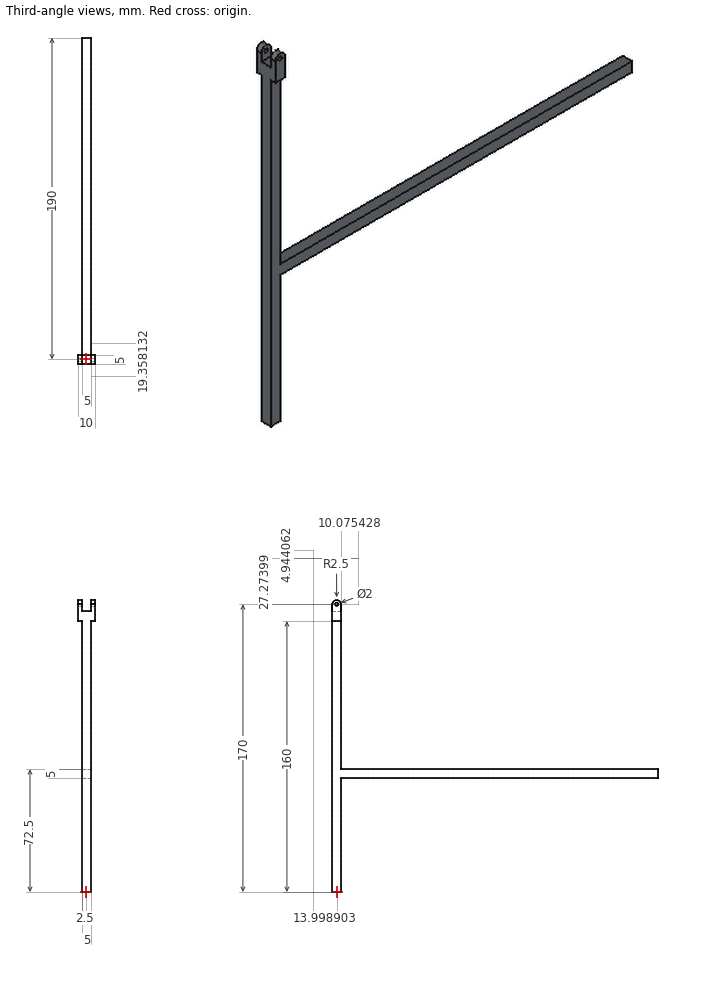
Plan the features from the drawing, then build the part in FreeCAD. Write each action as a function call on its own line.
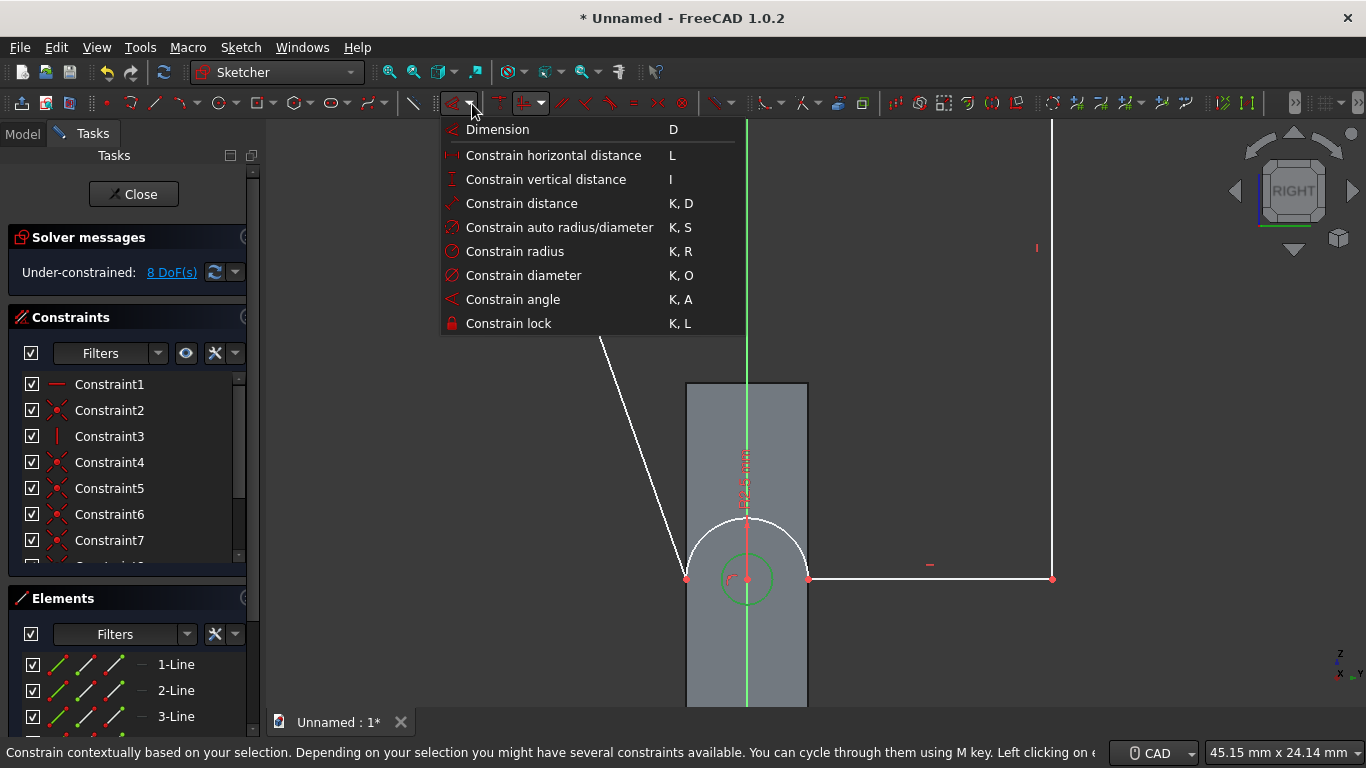
click(593, 275)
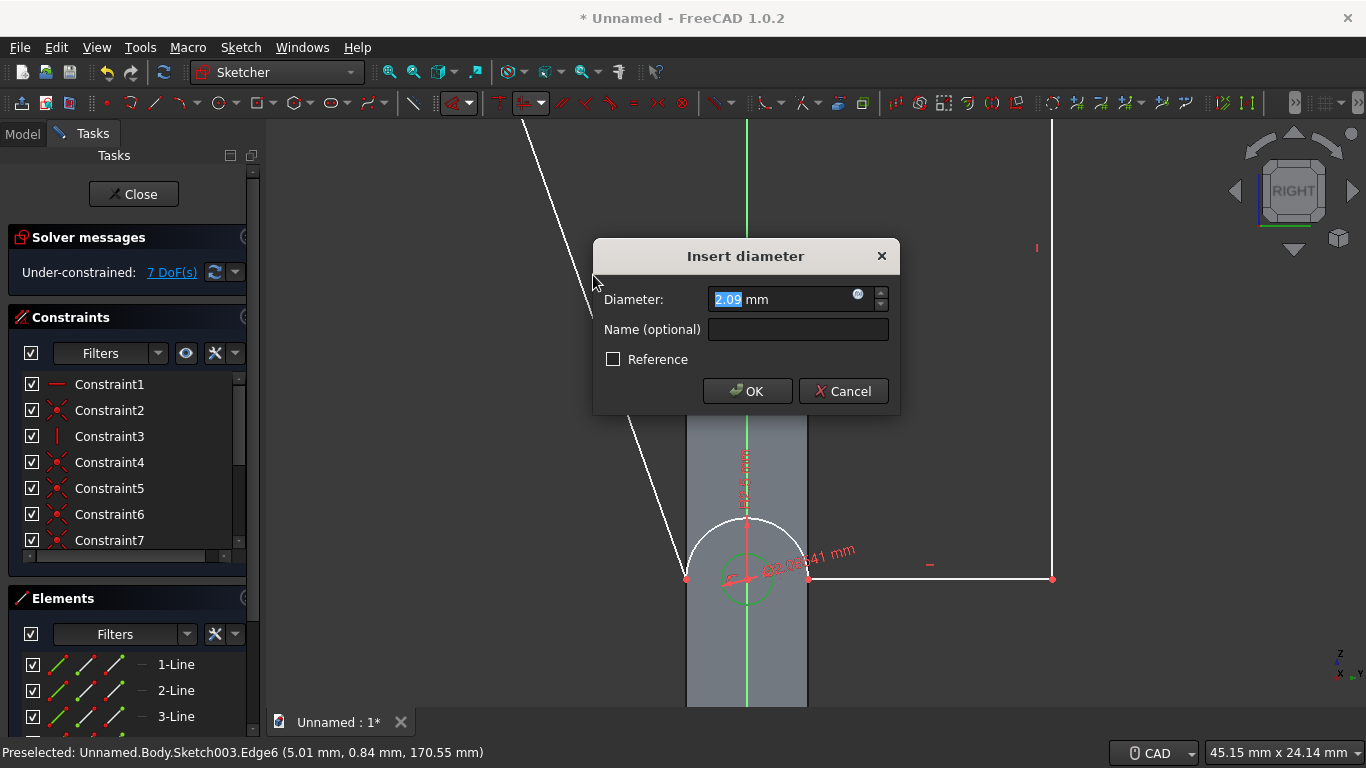
text(2)
key(Return)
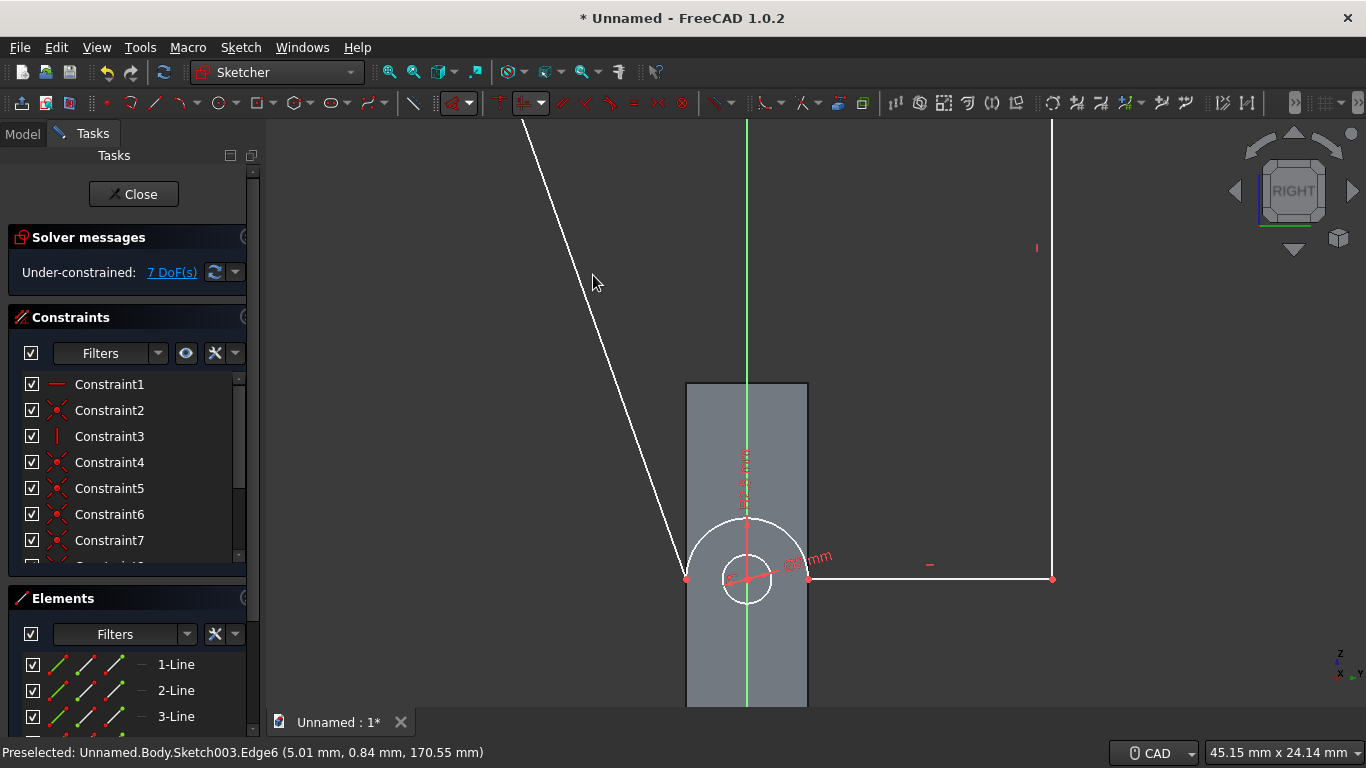
click(747, 579)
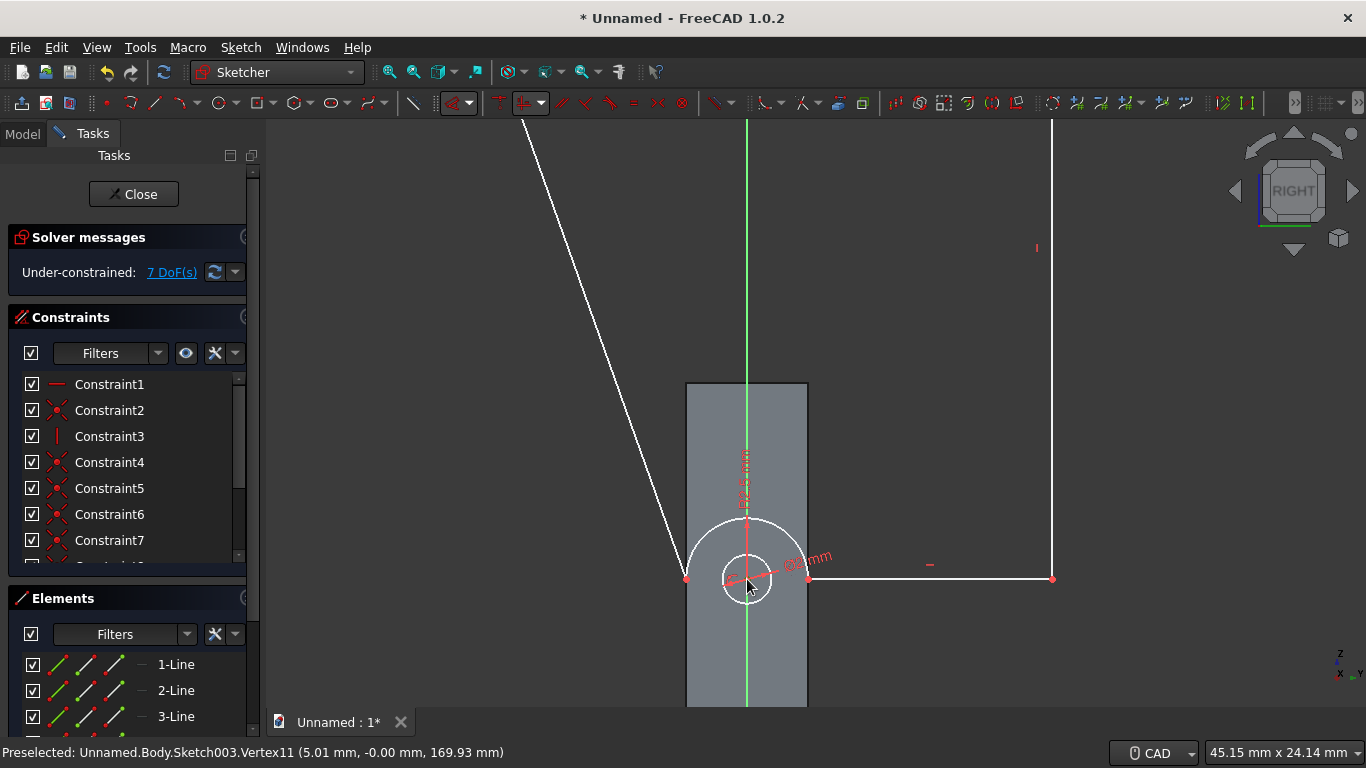
click(472, 104)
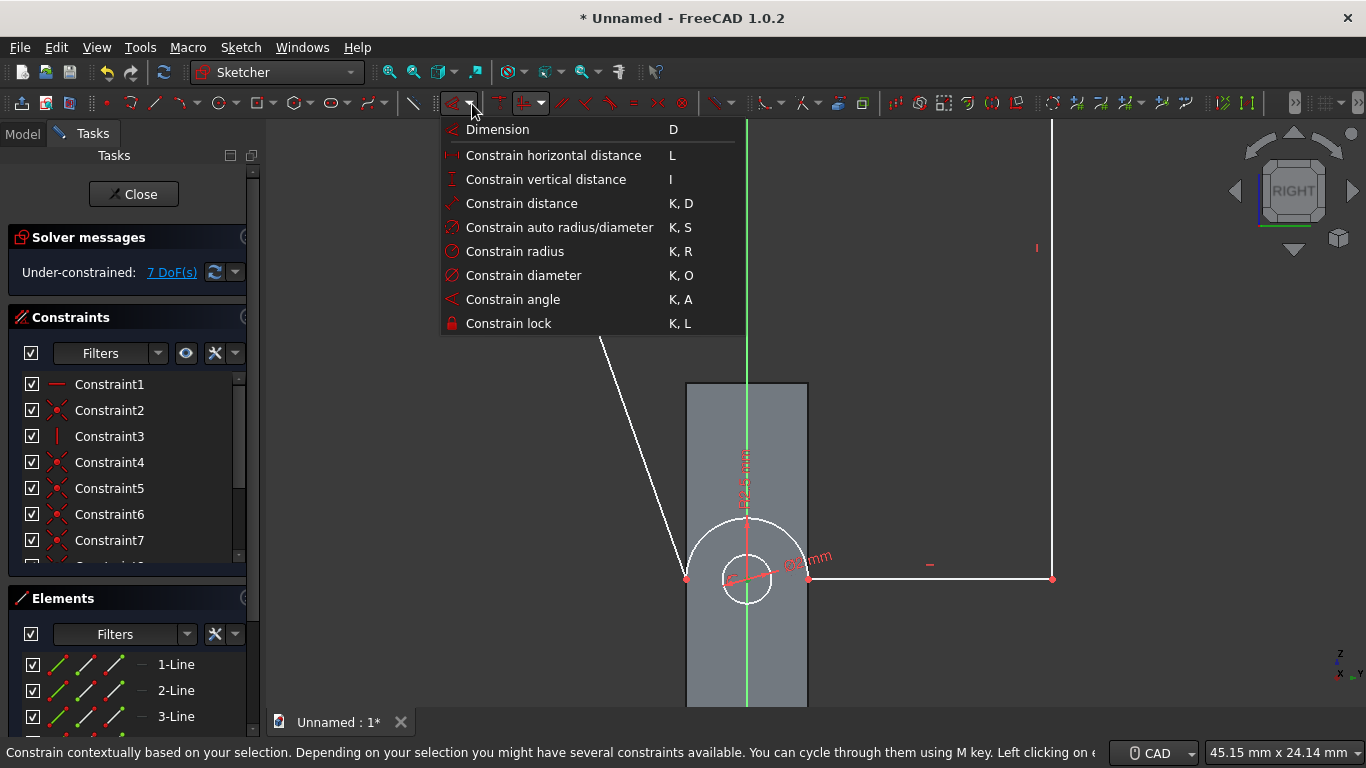
click(593, 179)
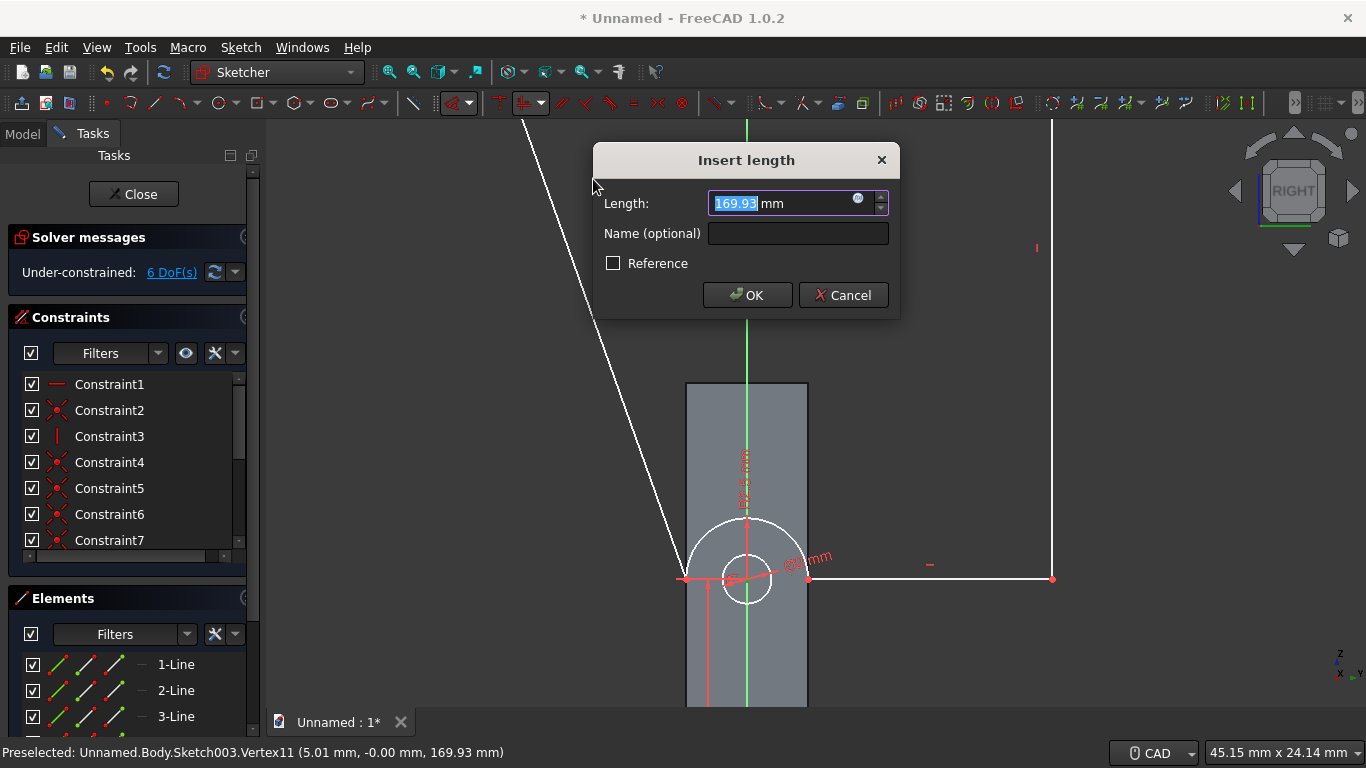
text(170)
key(Return)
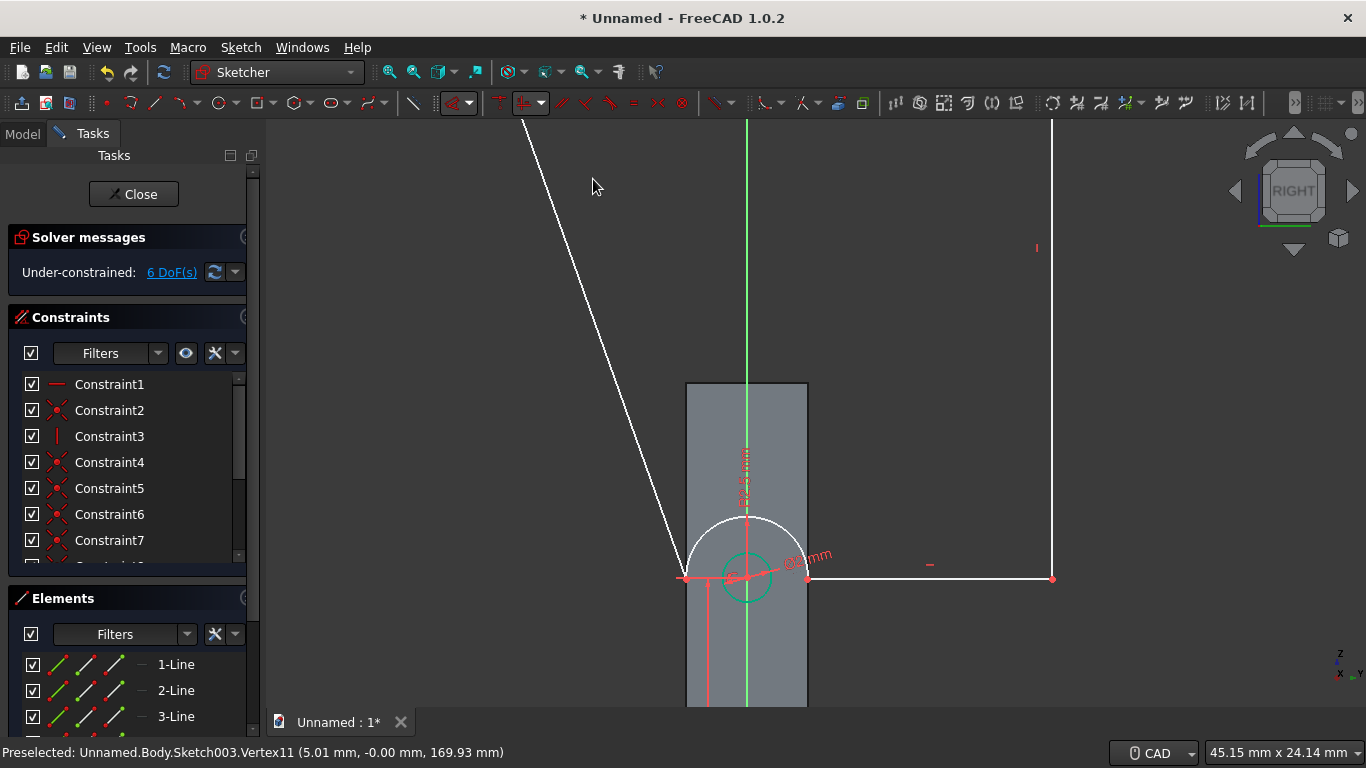
click(808, 579)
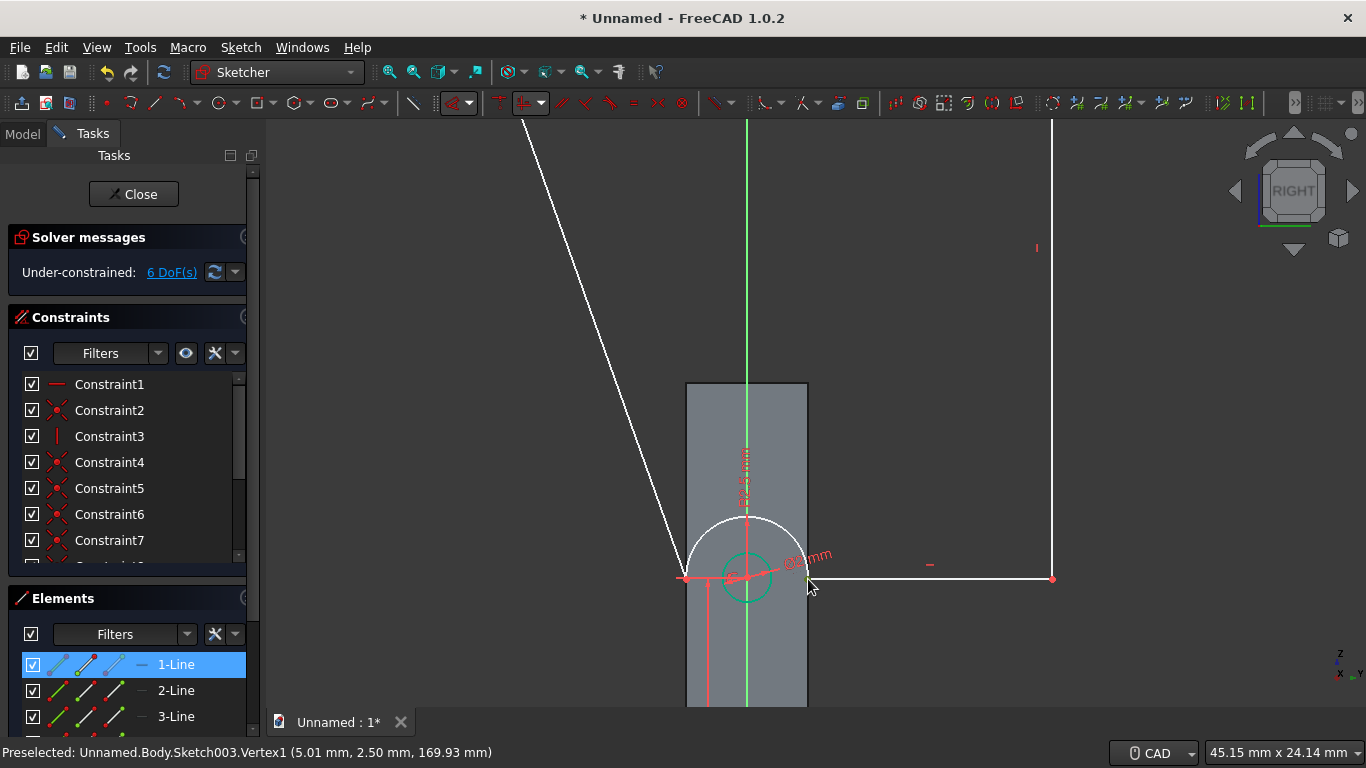
click(472, 104)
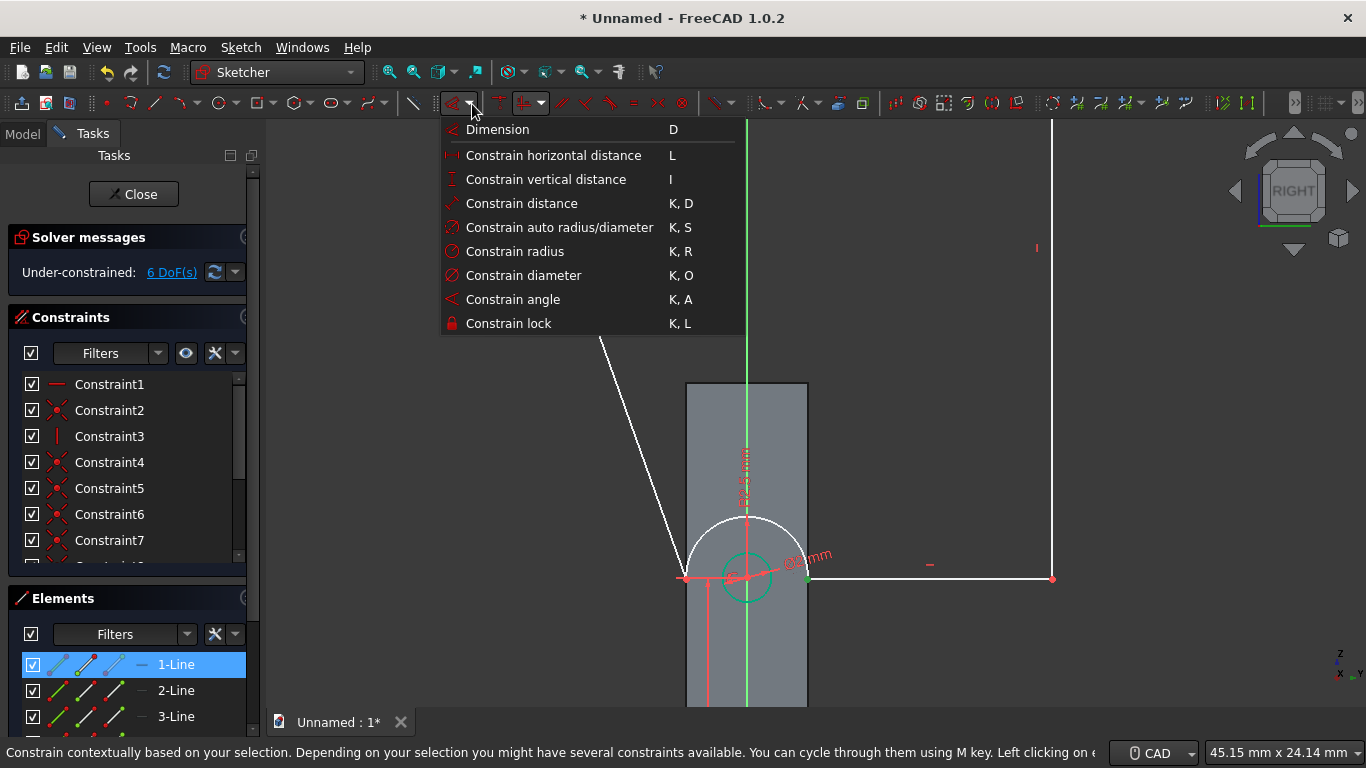
click(593, 179)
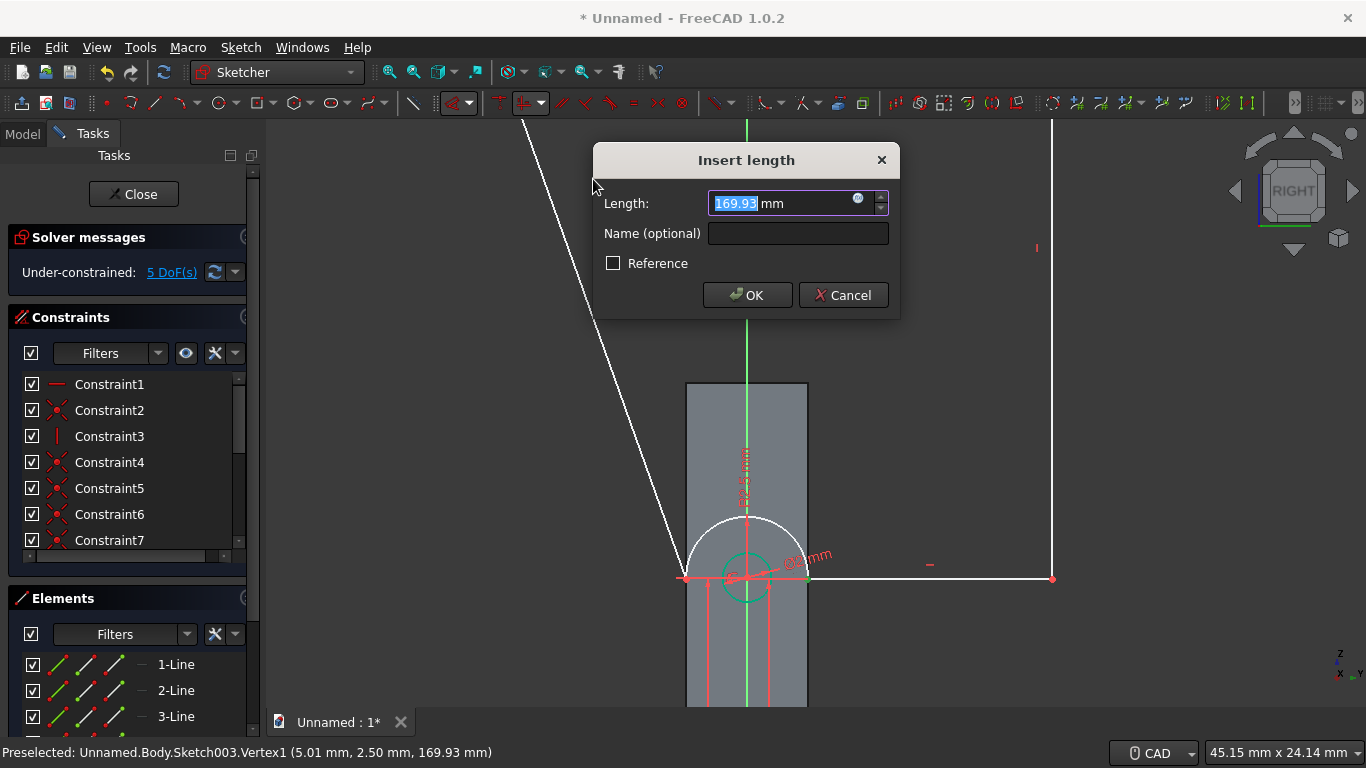
text(170)
key(Return)